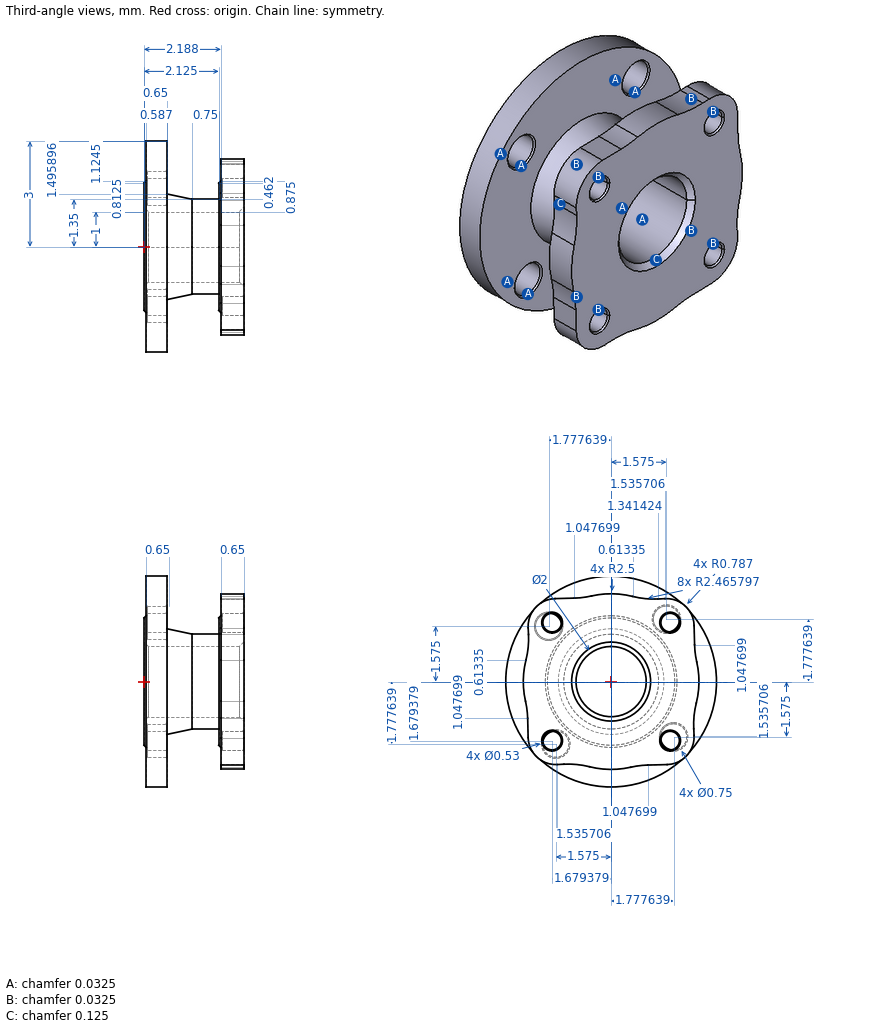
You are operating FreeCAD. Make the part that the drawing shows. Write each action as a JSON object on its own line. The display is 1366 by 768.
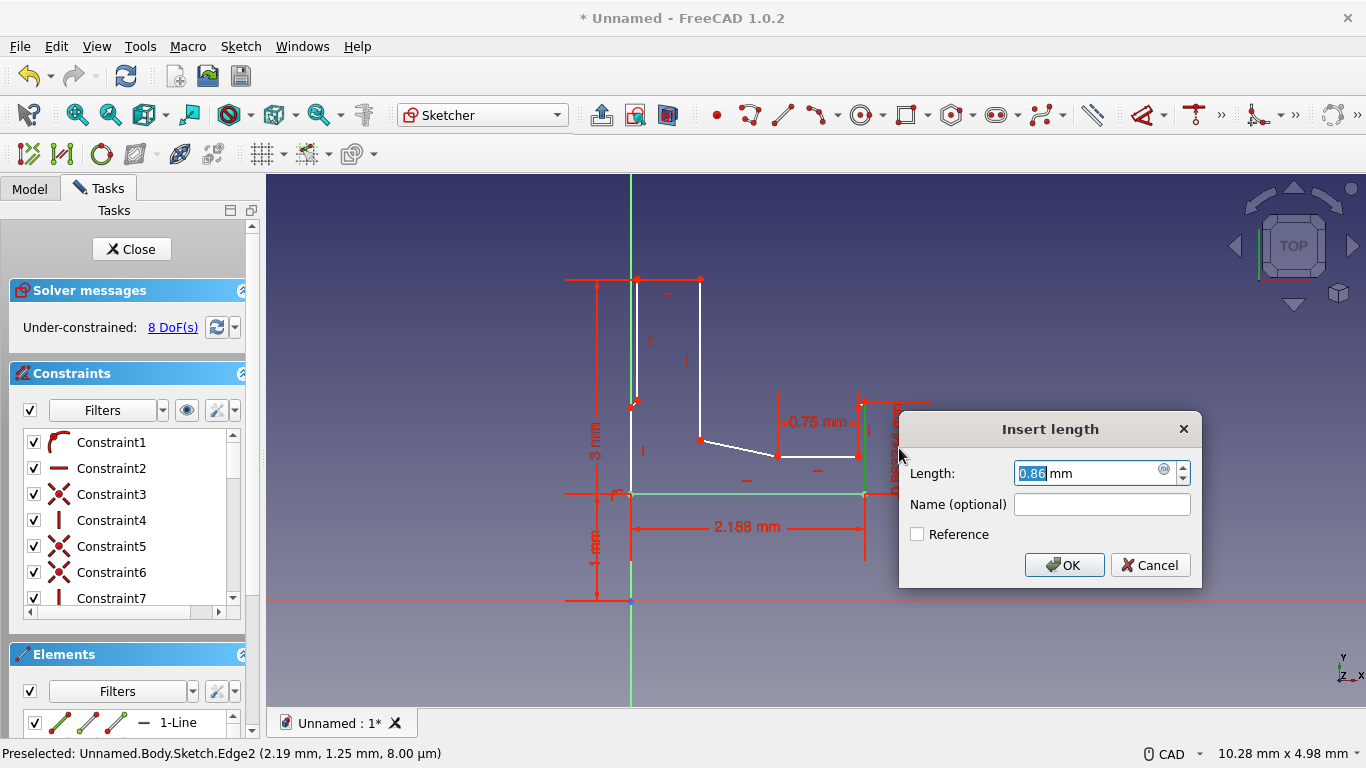
{"action": "type", "text": "0.875"}
{"action": "key", "text": "Return"}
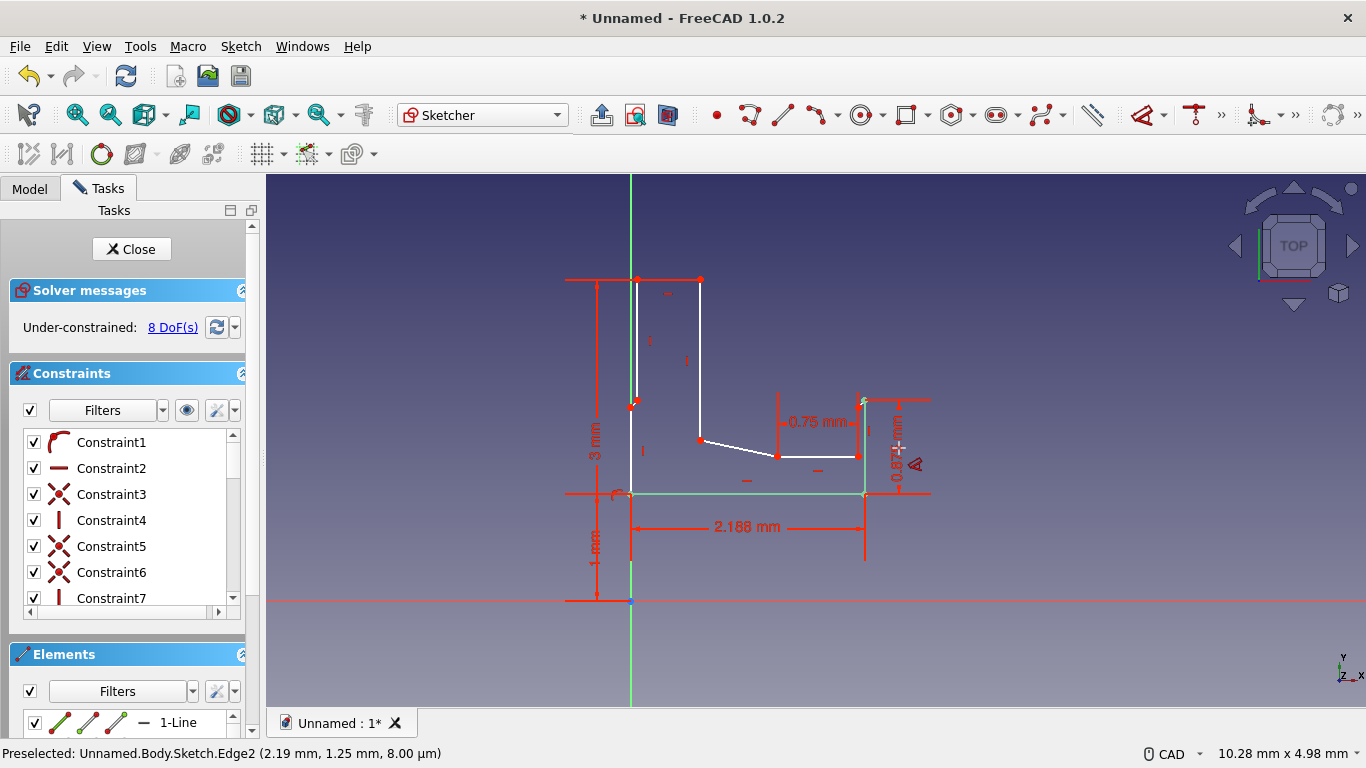
{"action": "scroll", "coordinate": [858, 422], "scroll_direction": "up", "scroll_amount": 4}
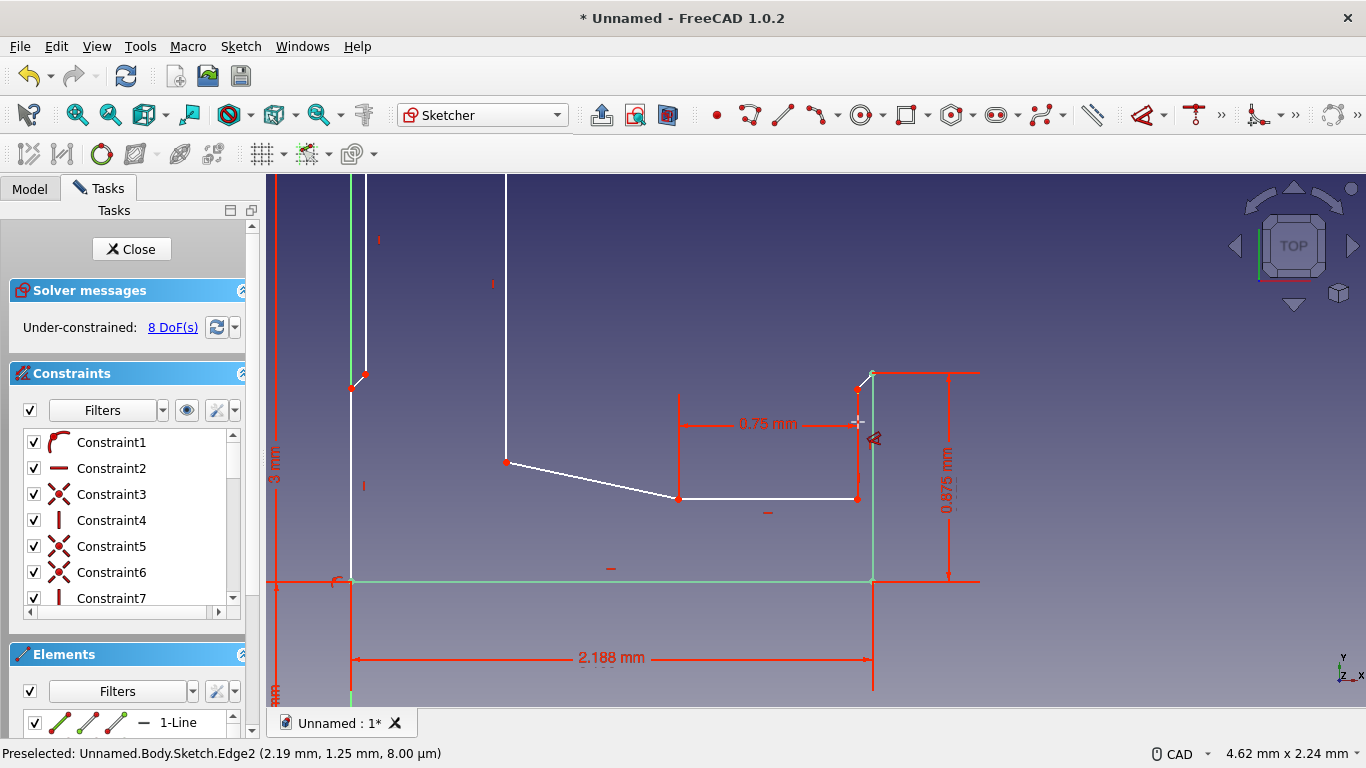
{"action": "left_click", "coordinate": [858, 422]}
{"action": "left_click", "coordinate": [892, 444]}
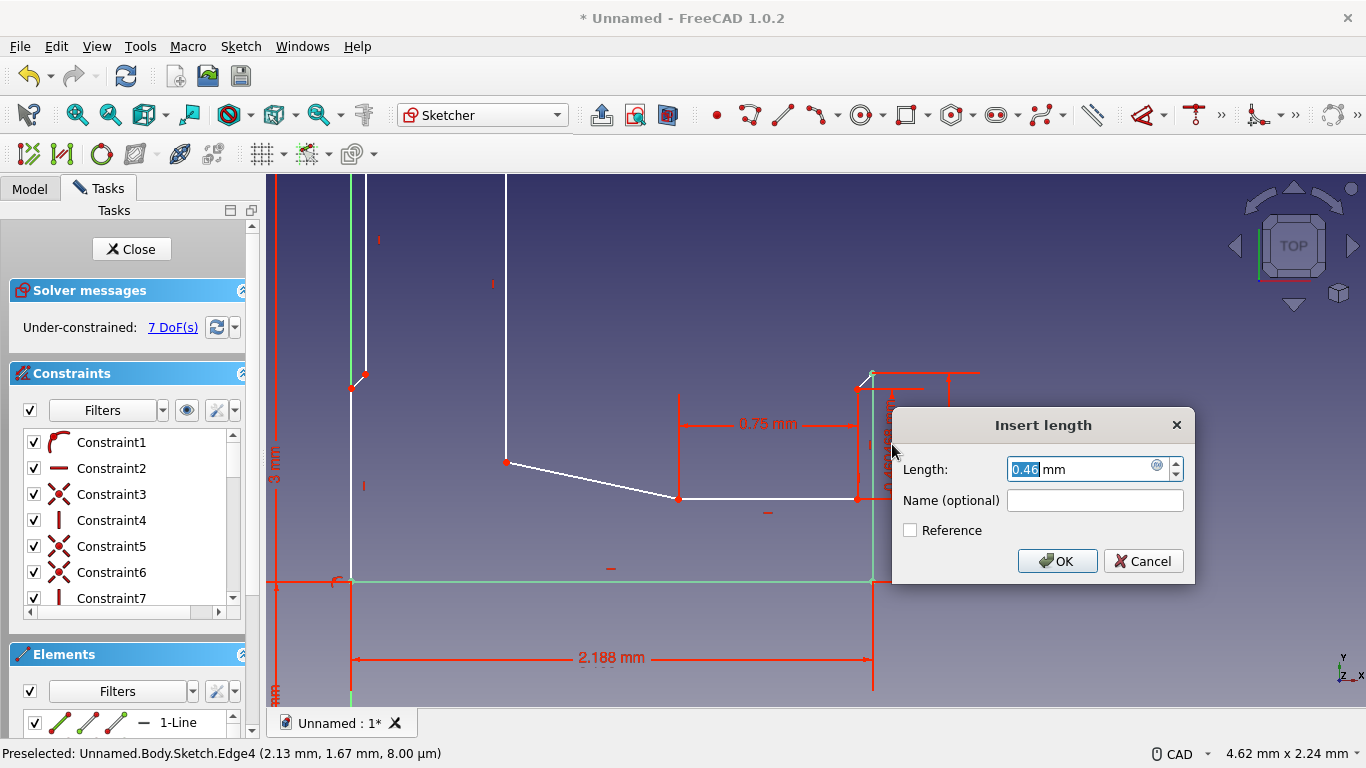
{"action": "type", "text": "0.462"}
{"action": "key", "text": "Return"}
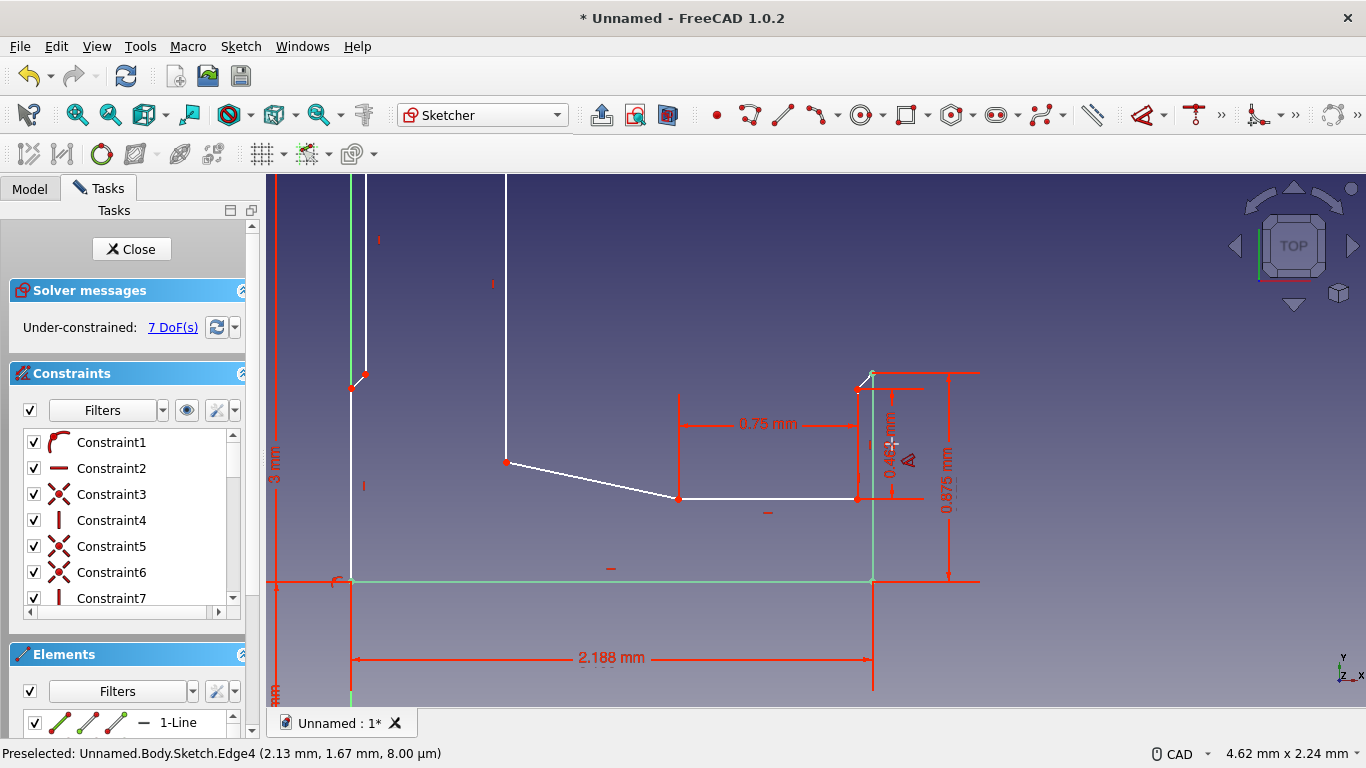
{"action": "scroll", "coordinate": [858, 422], "scroll_direction": "down", "scroll_amount": 4}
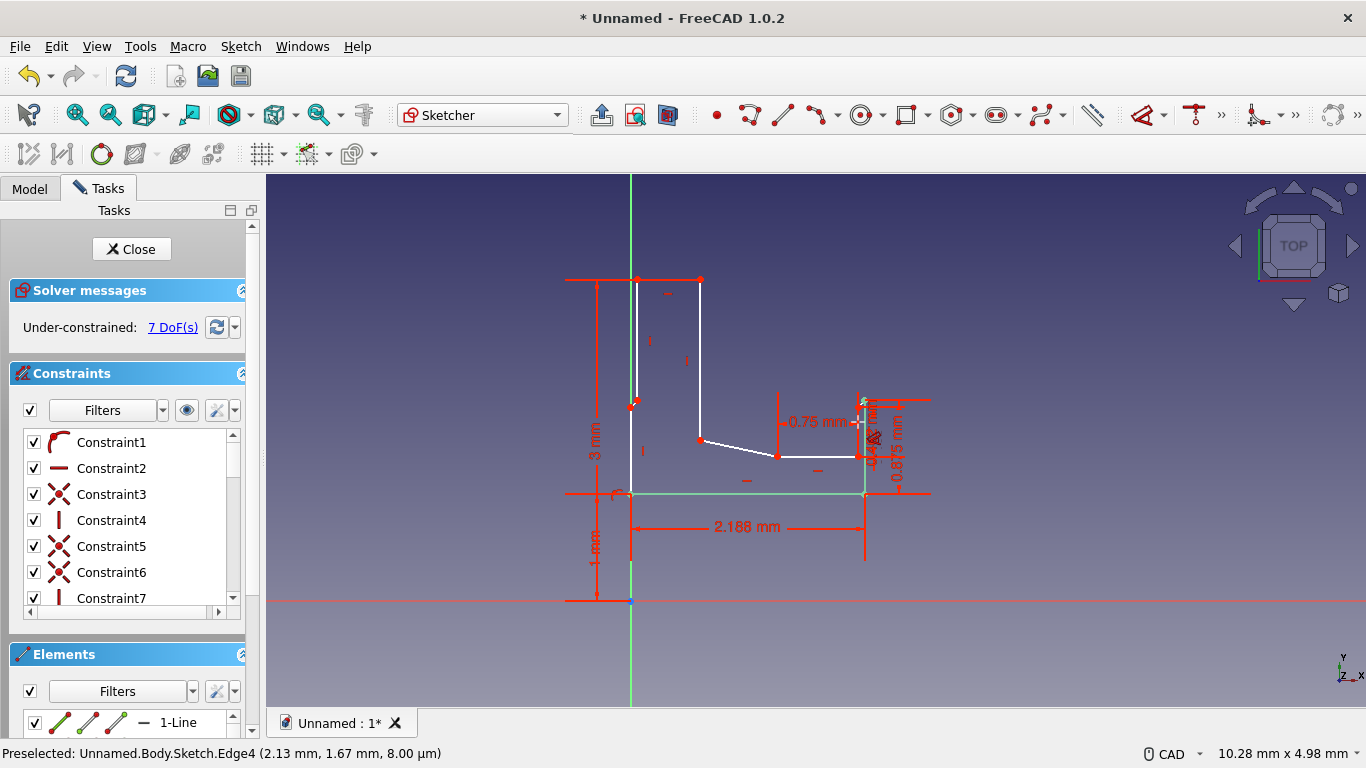
{"action": "left_click", "coordinate": [681, 280]}
{"action": "left_click", "coordinate": [669, 246]}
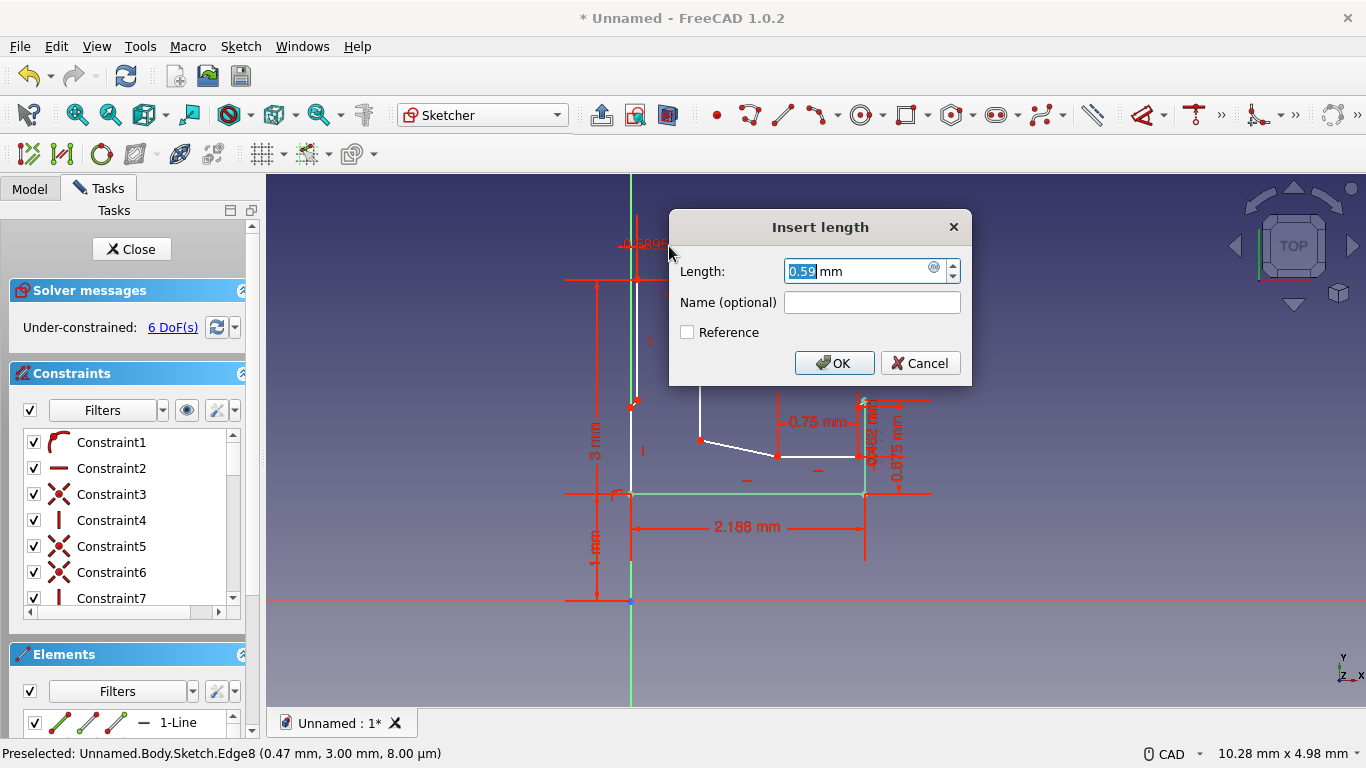
{"action": "type", "text": "0.587"}
{"action": "key", "text": "Return"}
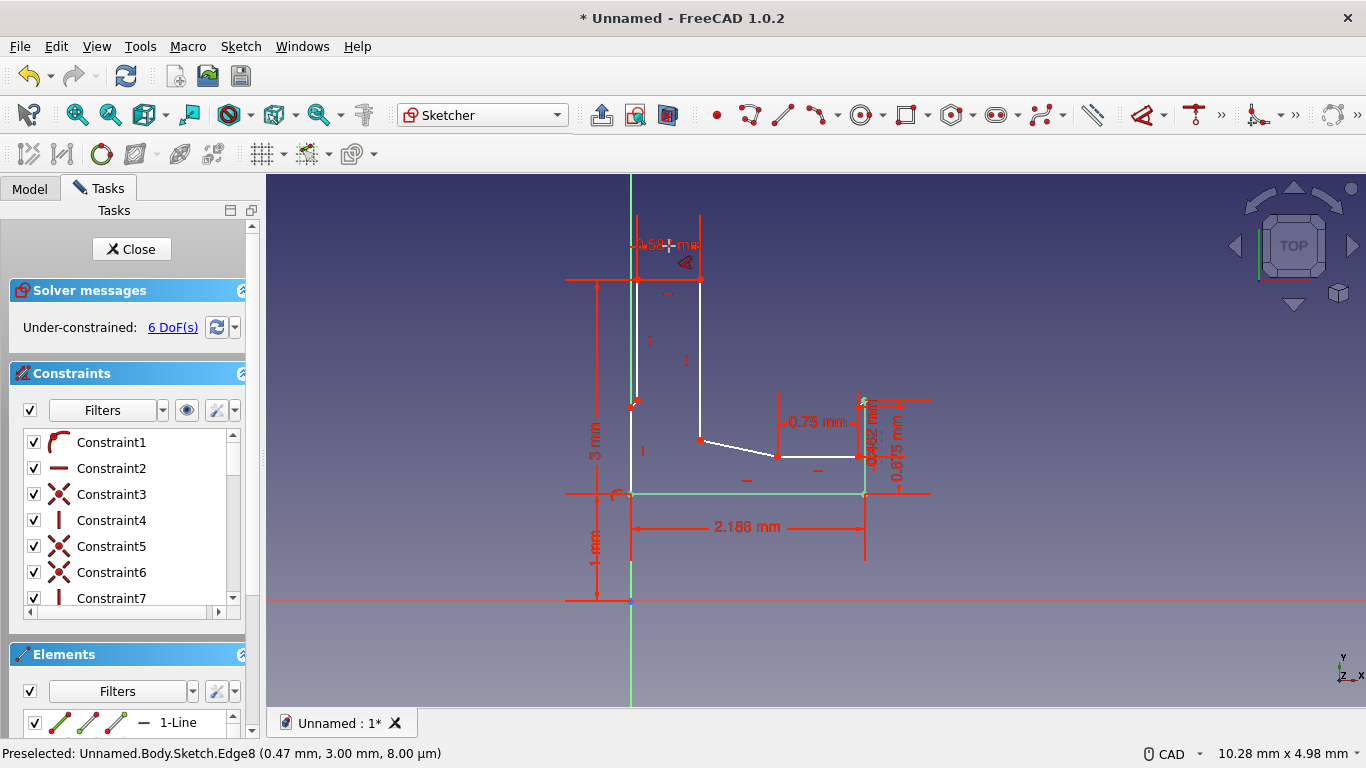
{"action": "left_click", "coordinate": [858, 457]}
{"action": "left_click", "coordinate": [597, 496]}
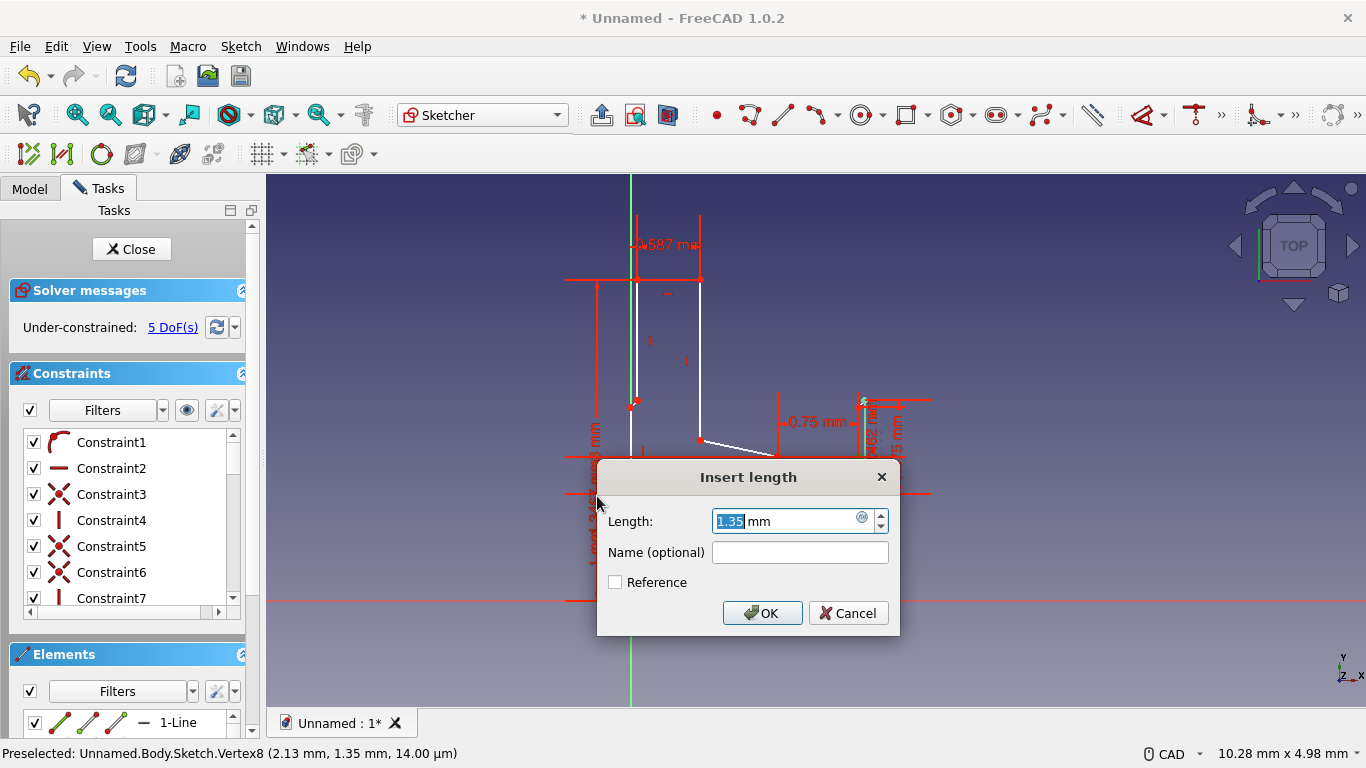
{"action": "type", "text": "1.35"}
{"action": "key", "text": "Return"}